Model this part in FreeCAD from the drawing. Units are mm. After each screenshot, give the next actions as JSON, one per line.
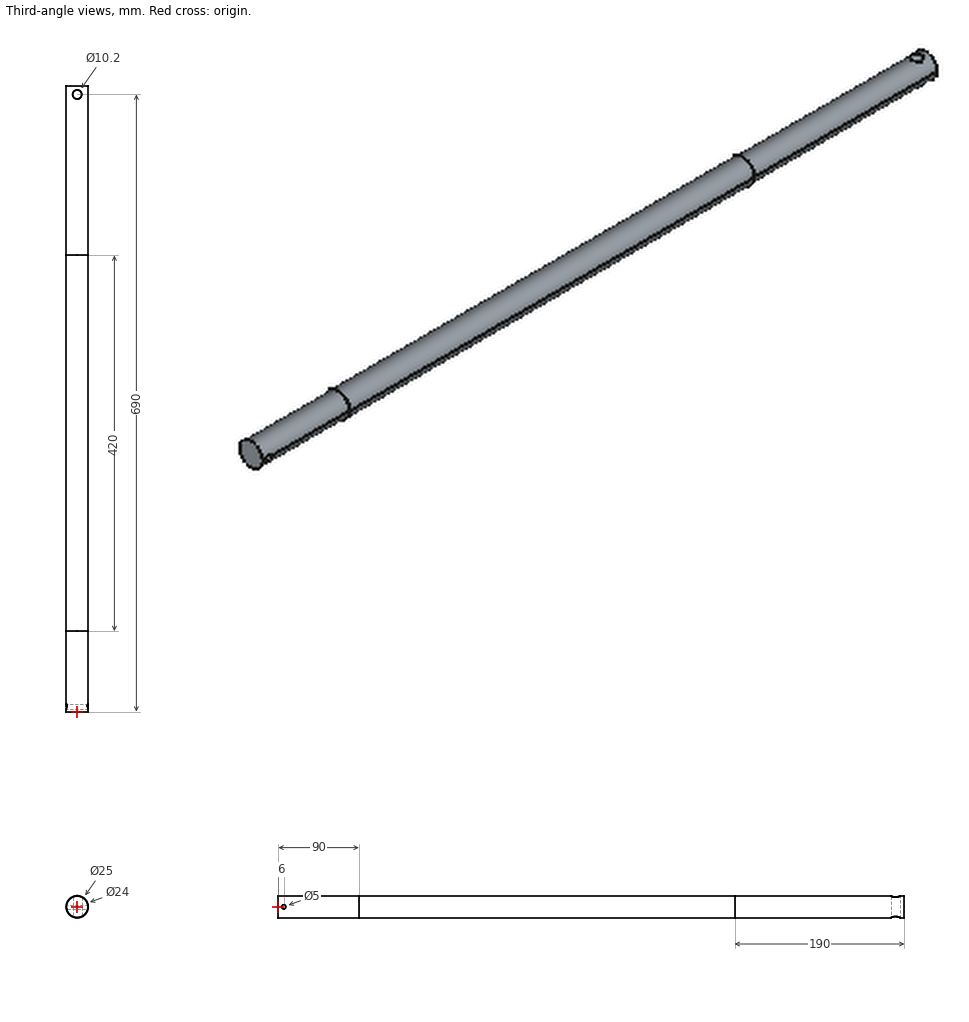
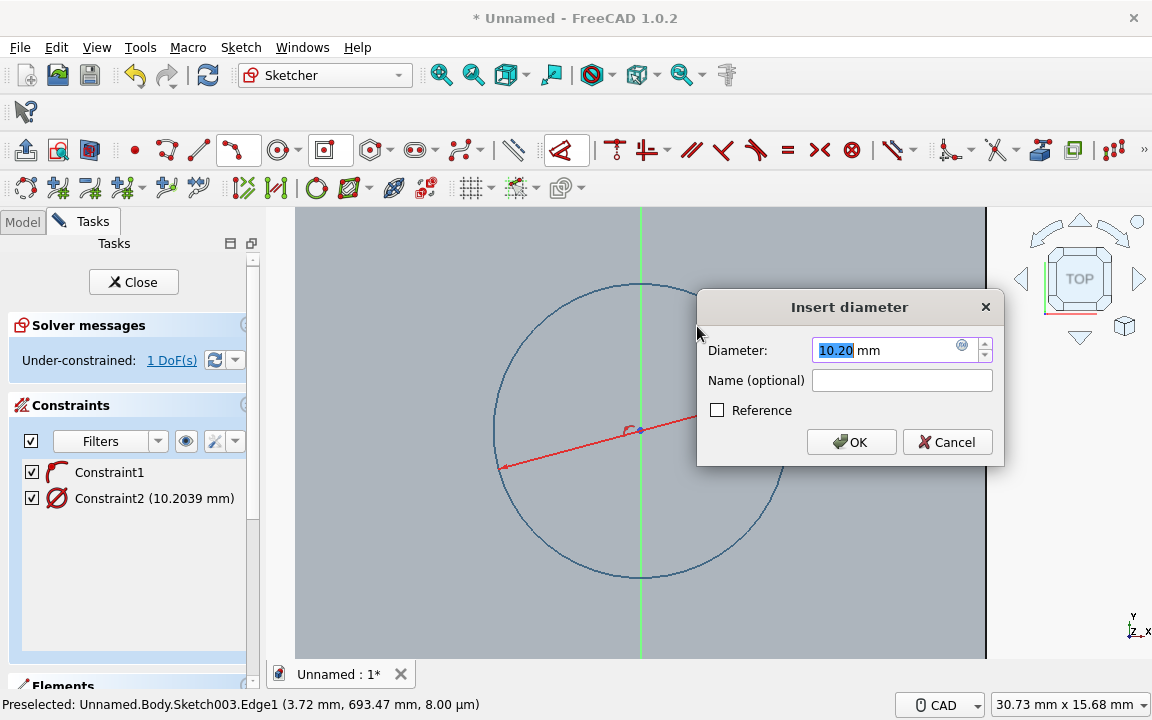
{"action": "type", "text": "10.2"}
{"action": "key", "text": "Return"}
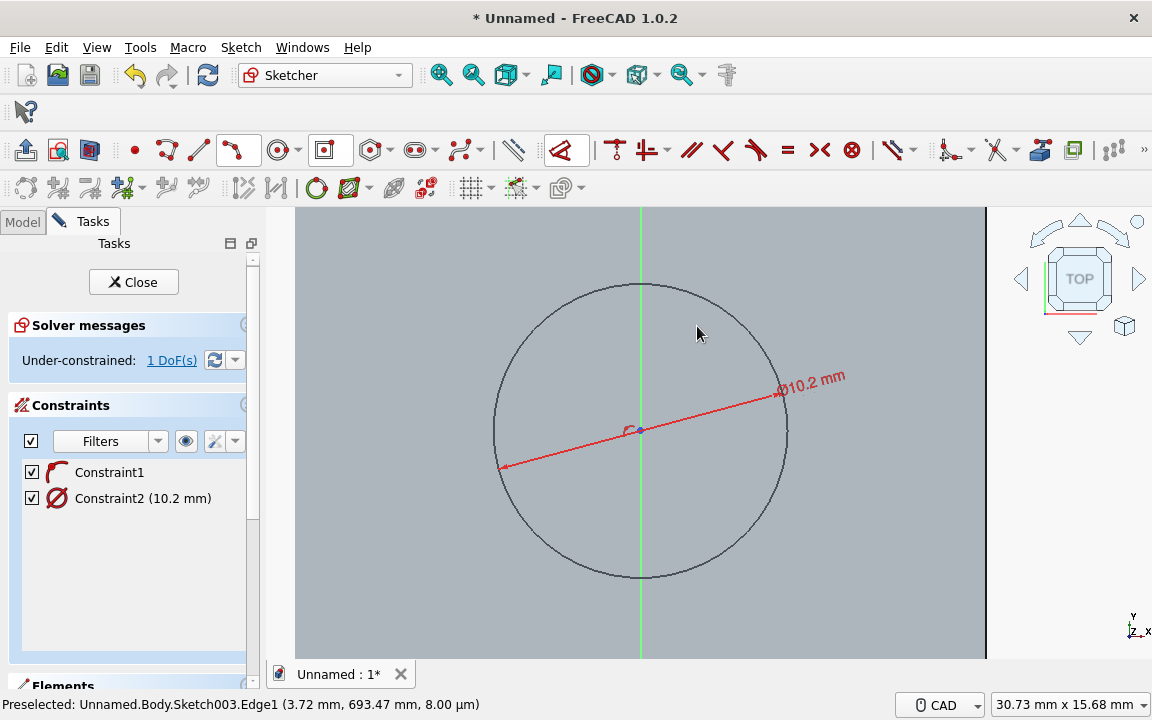
{"action": "left_click", "coordinate": [641, 431]}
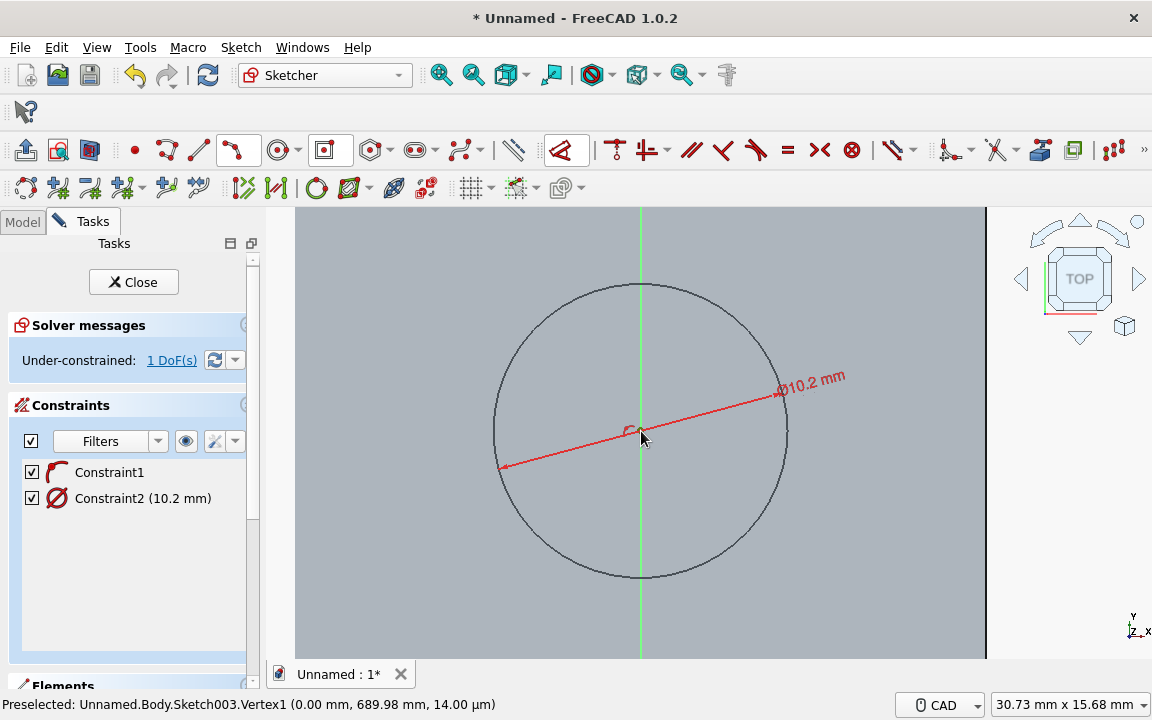
{"action": "key", "text": "i"}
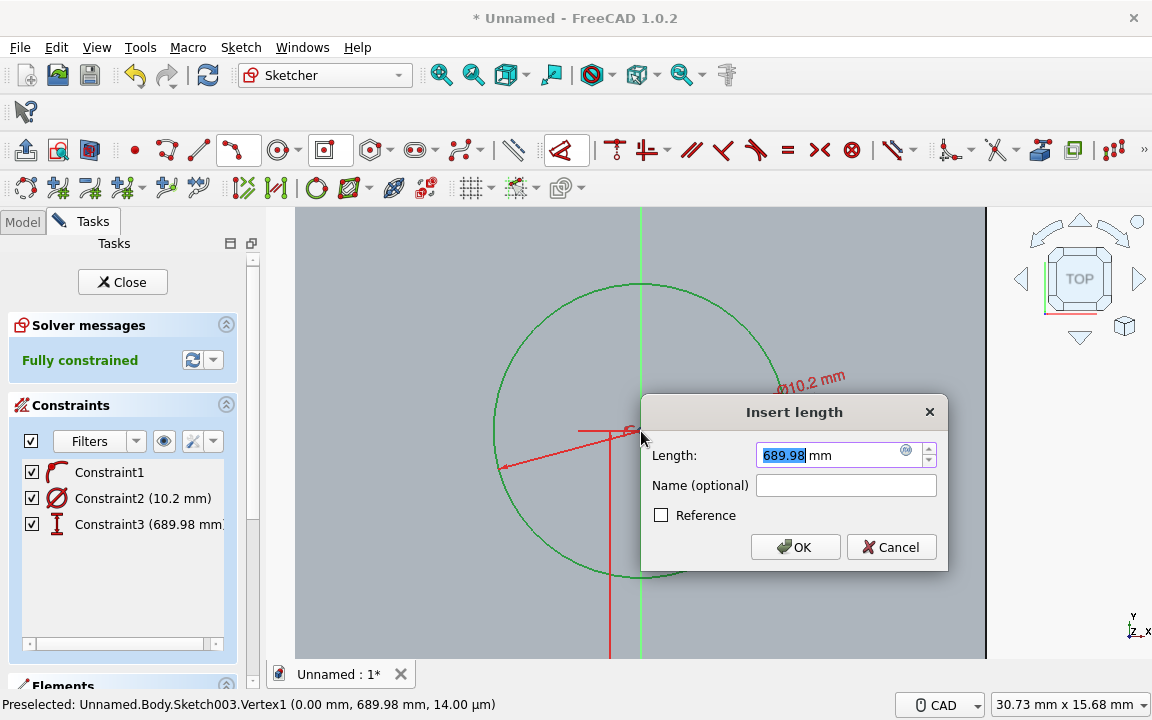
{"action": "type", "text": "690"}
{"action": "key", "text": "Return"}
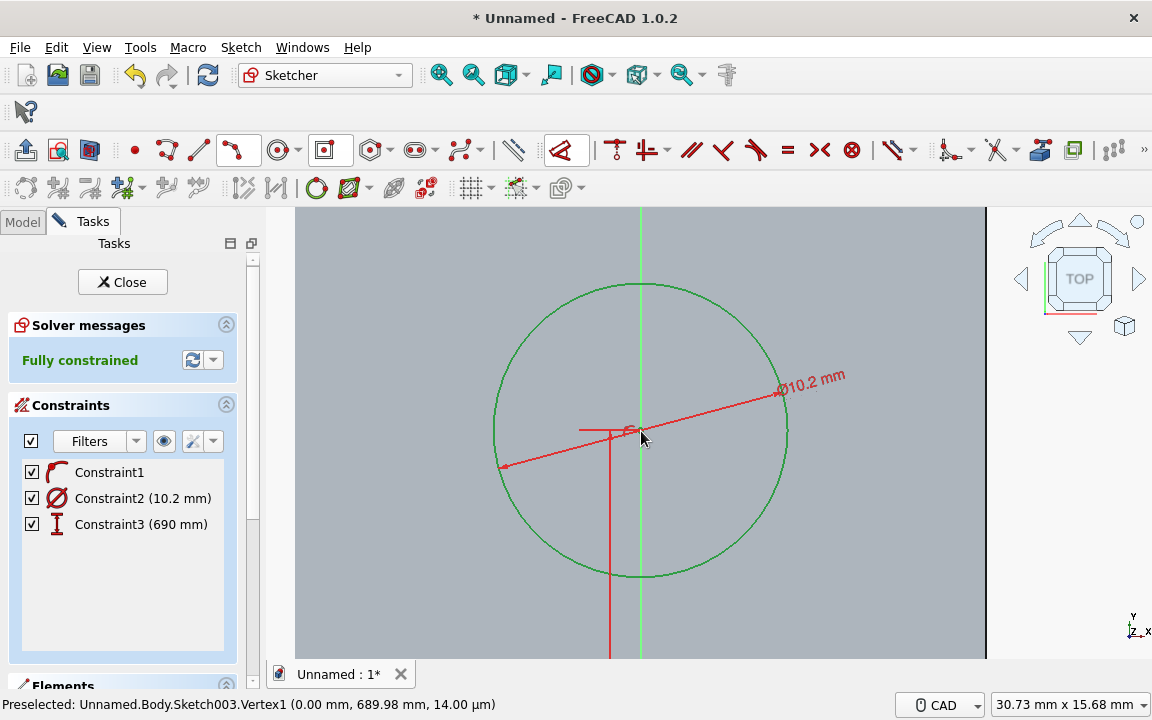
{"action": "left_click", "coordinate": [123, 282]}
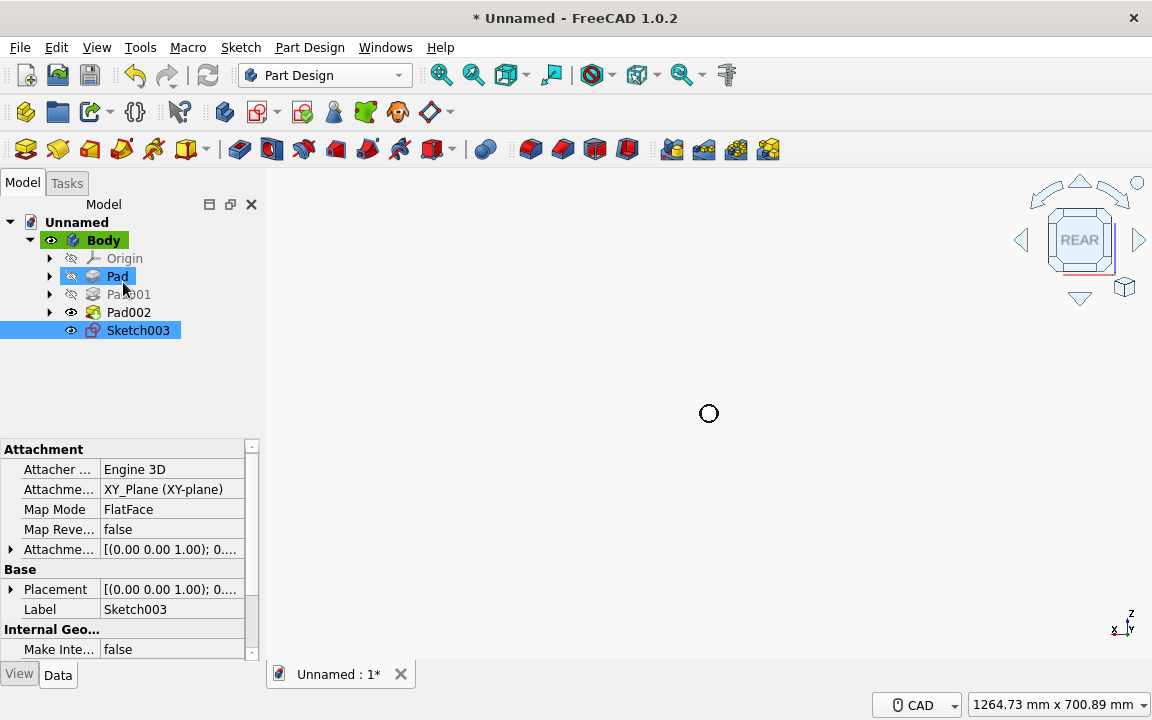
{"action": "left_click", "coordinate": [240, 150]}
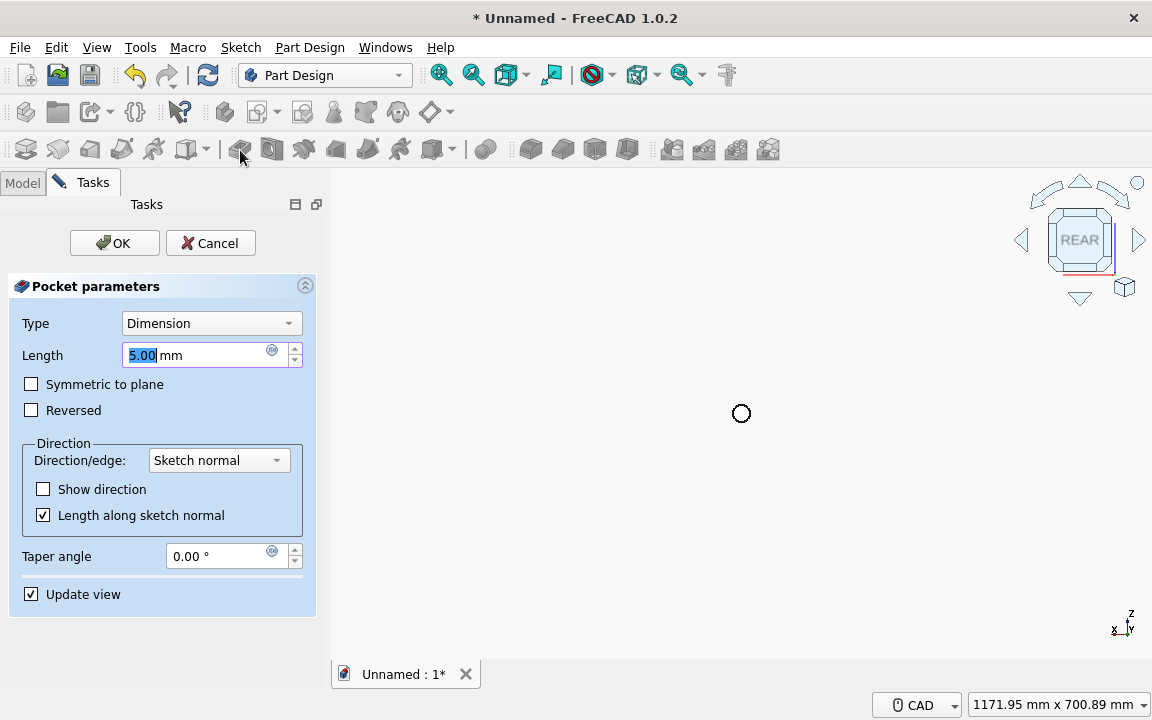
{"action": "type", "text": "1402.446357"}
{"action": "key", "text": "Tab"}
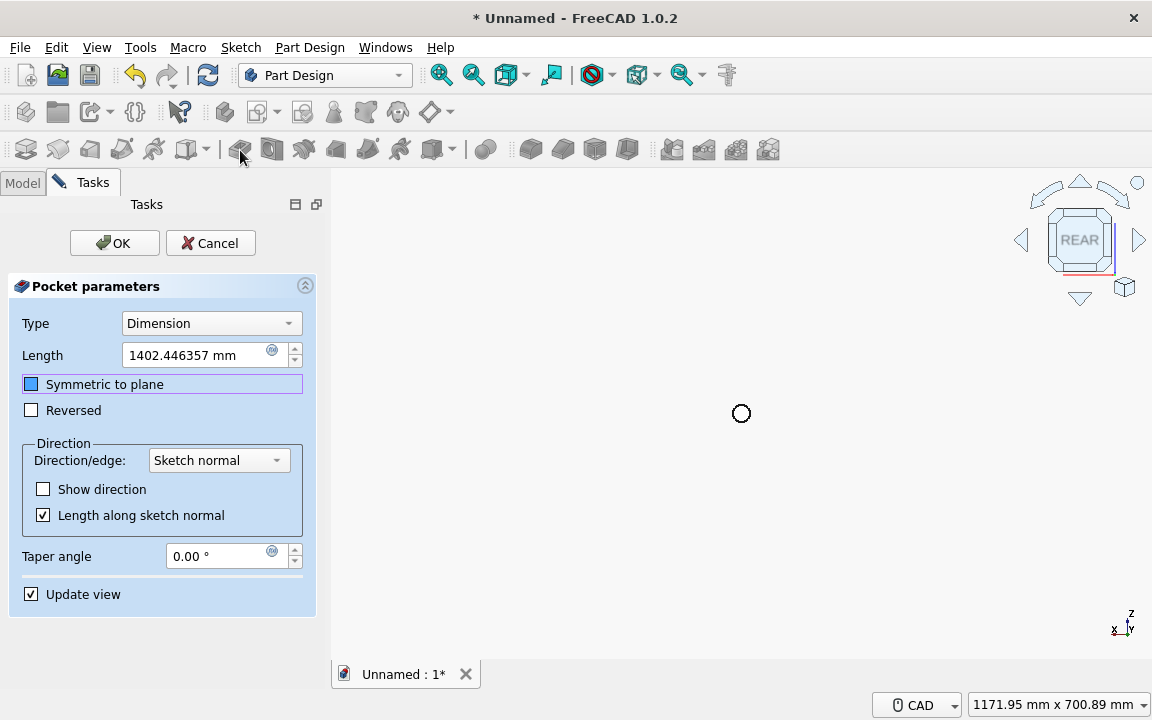
{"action": "left_click", "coordinate": [30, 384]}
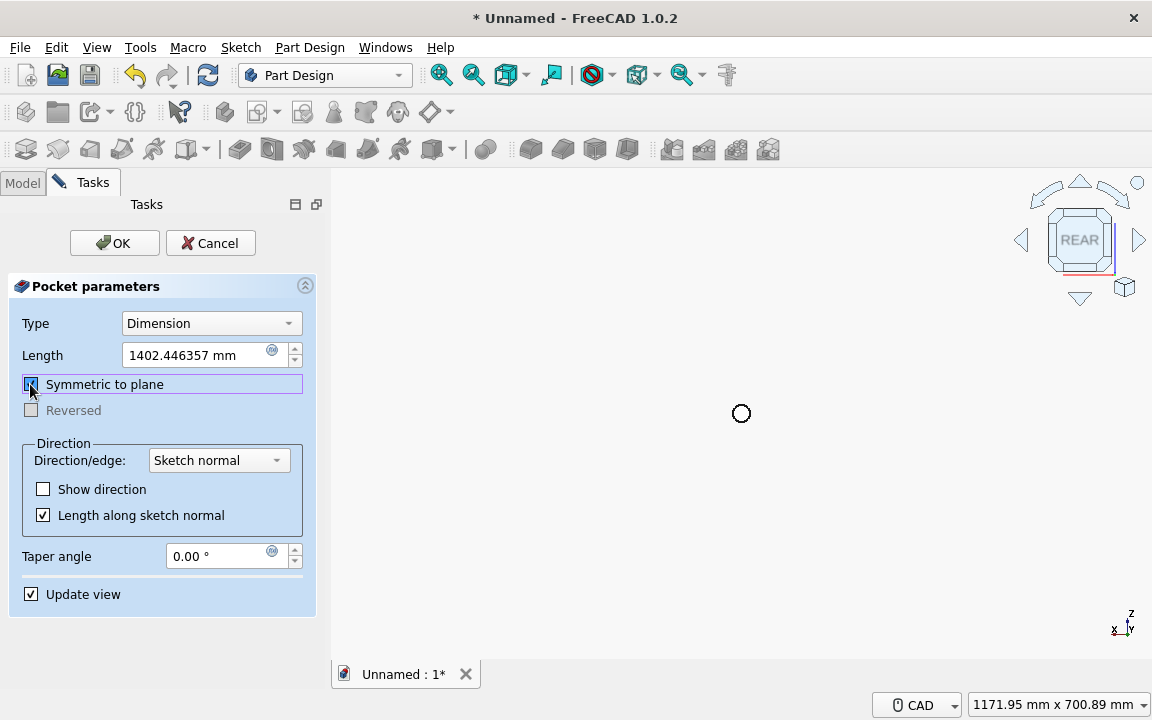
{"action": "left_click", "coordinate": [115, 243]}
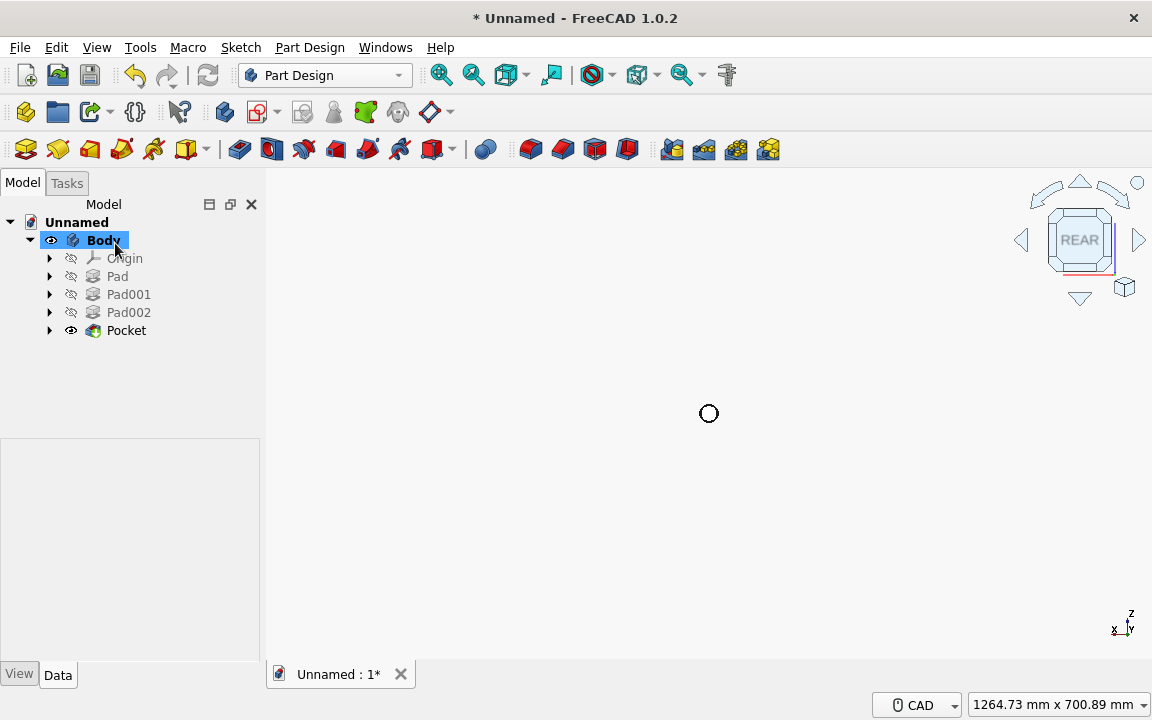
{"action": "key", "text": "v f"}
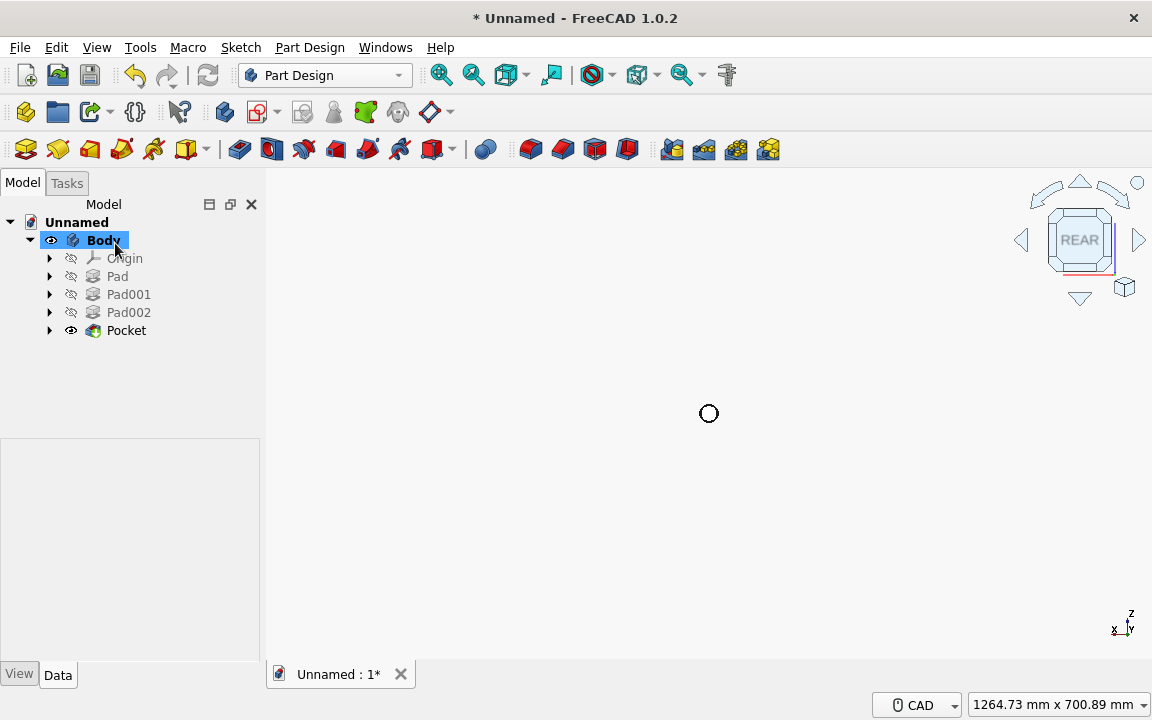
{"action": "left_click", "coordinate": [258, 112]}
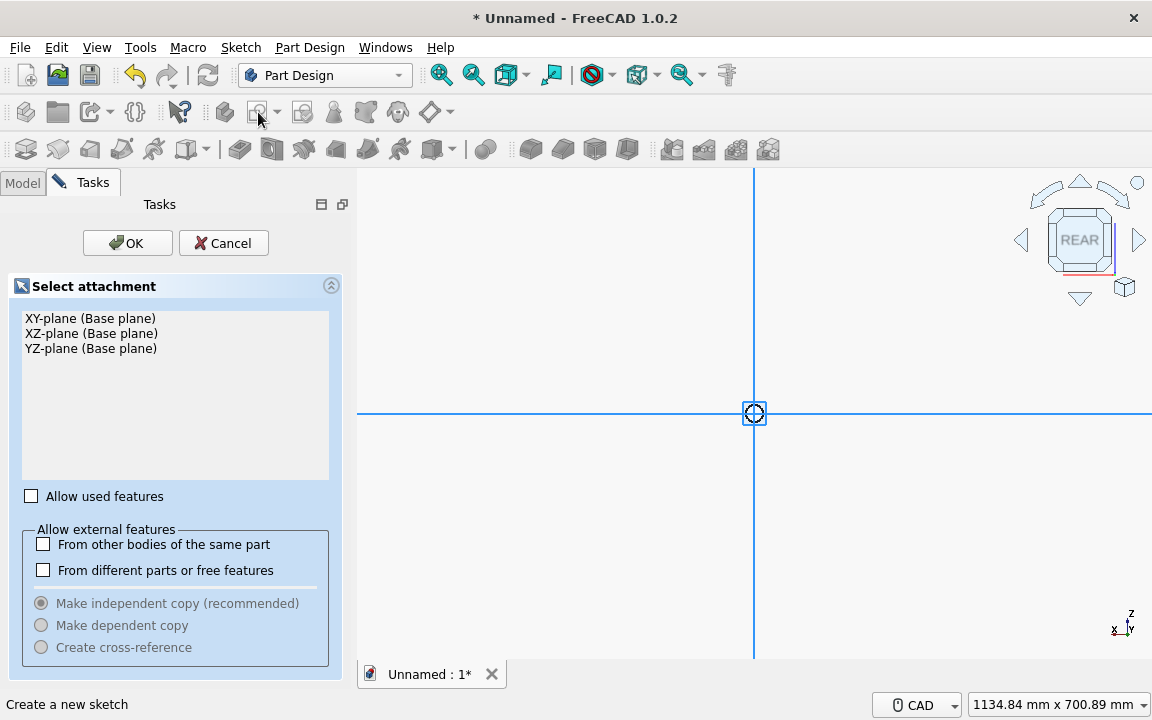
{"action": "left_click", "coordinate": [82, 348]}